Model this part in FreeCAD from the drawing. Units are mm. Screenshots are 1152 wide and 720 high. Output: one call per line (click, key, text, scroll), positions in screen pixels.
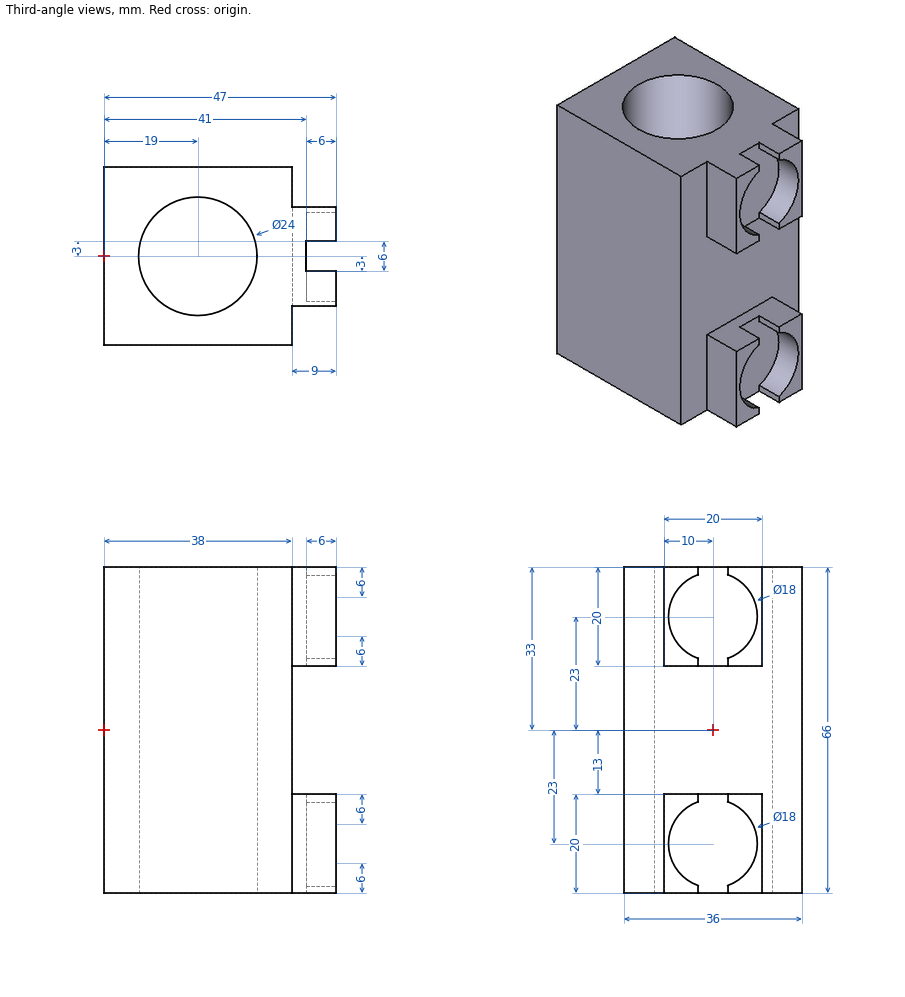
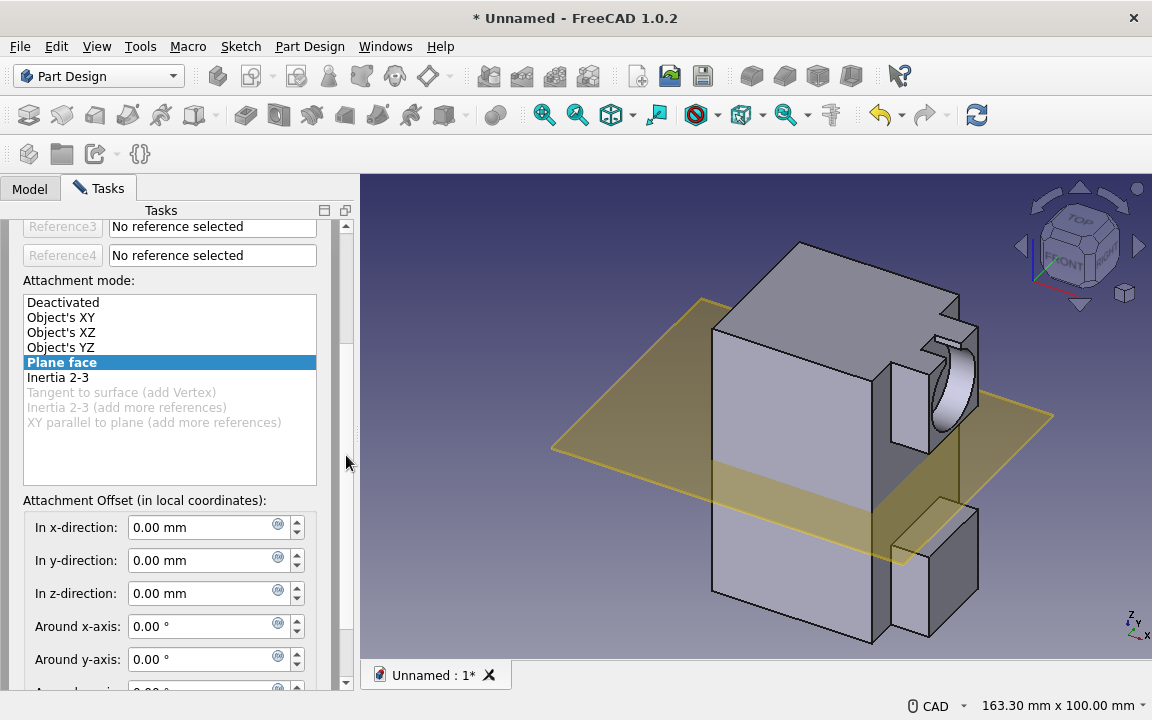
triple_click(210, 594)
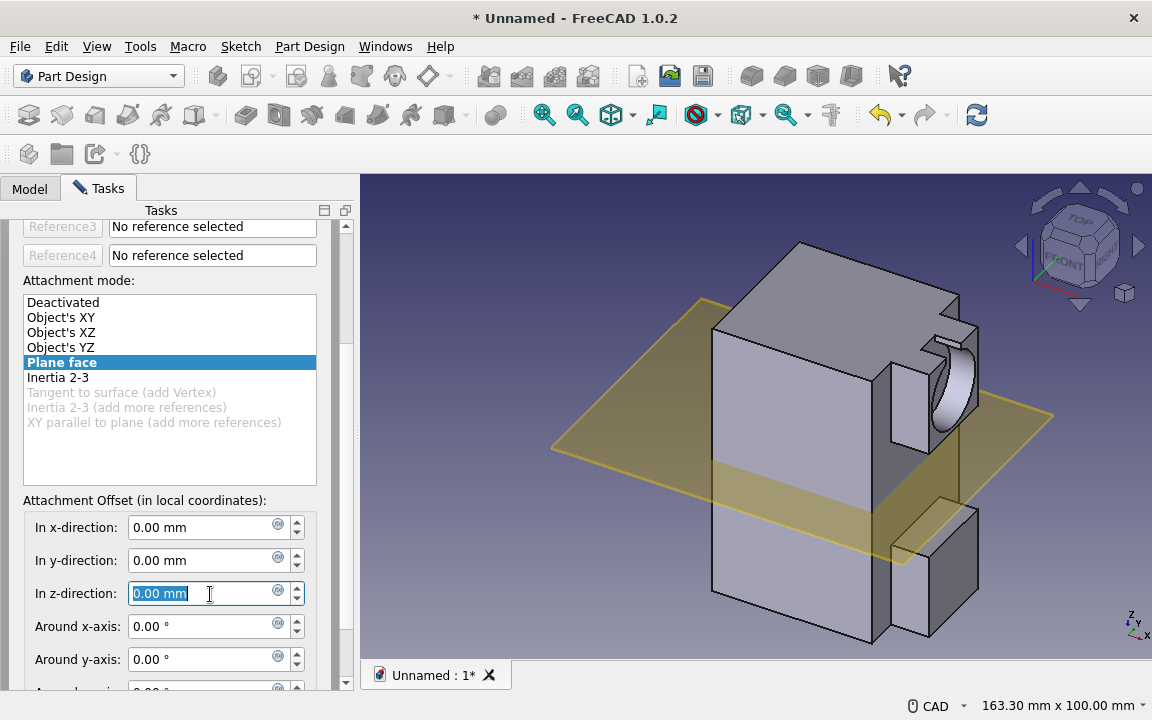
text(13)
key(Tab)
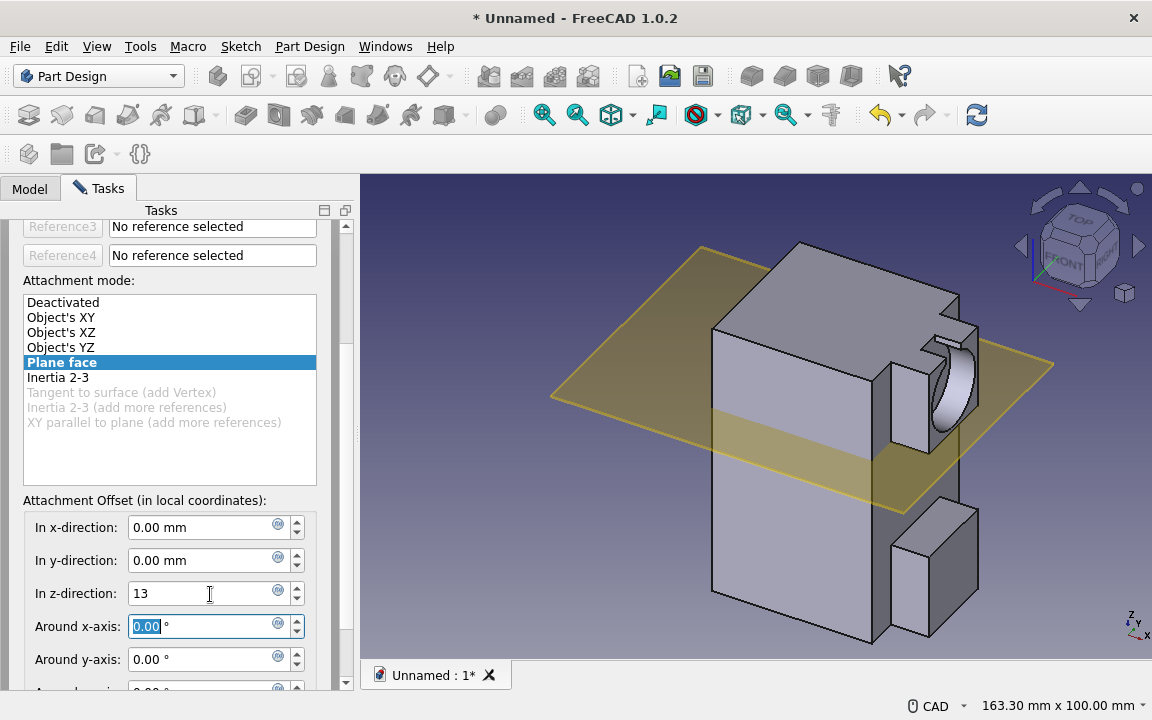
scroll(346, 455, up, 4)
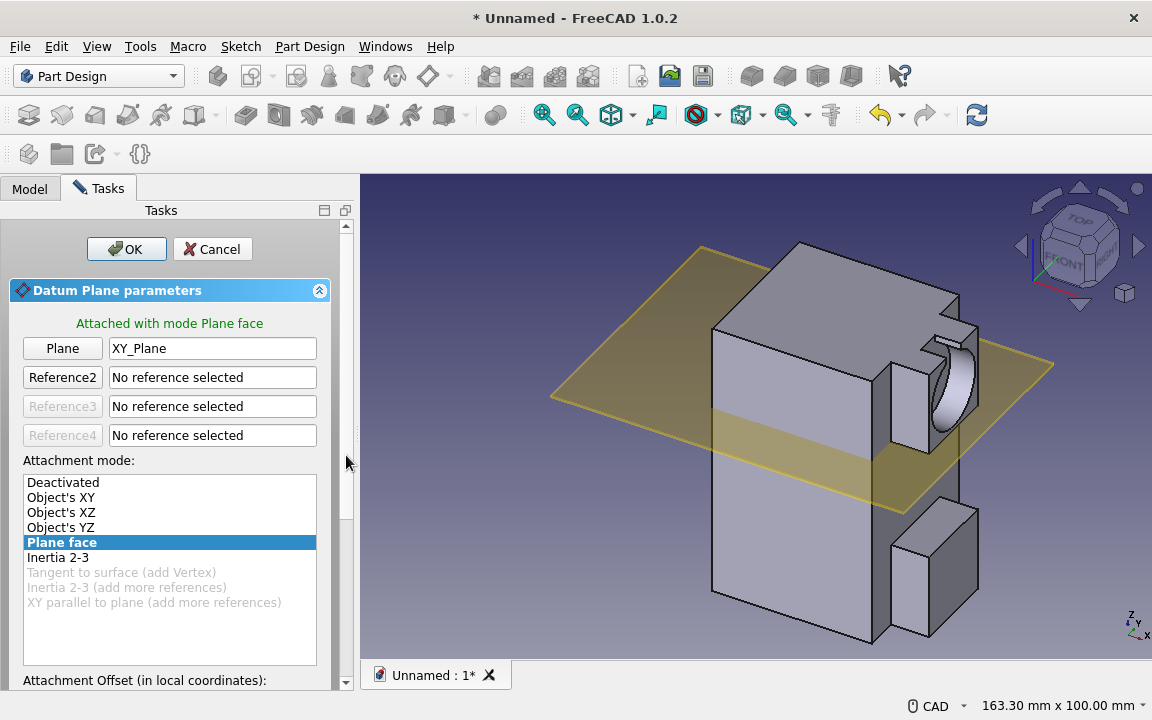
click(127, 249)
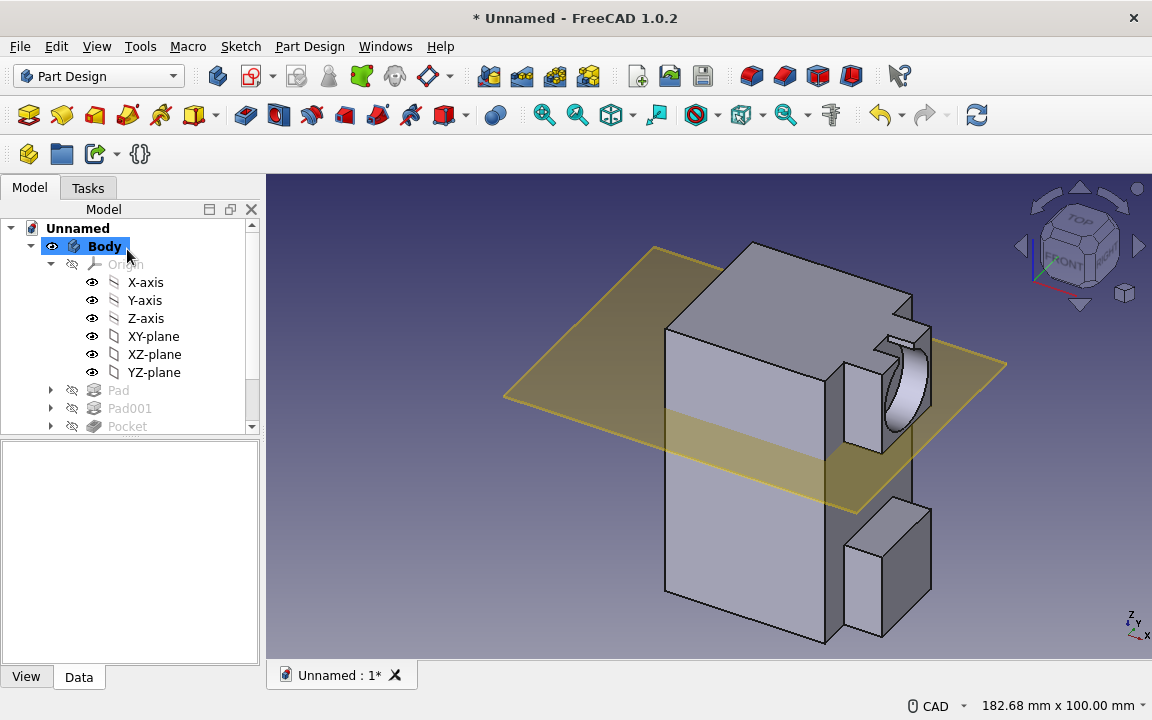
scroll(101, 332, down, 3)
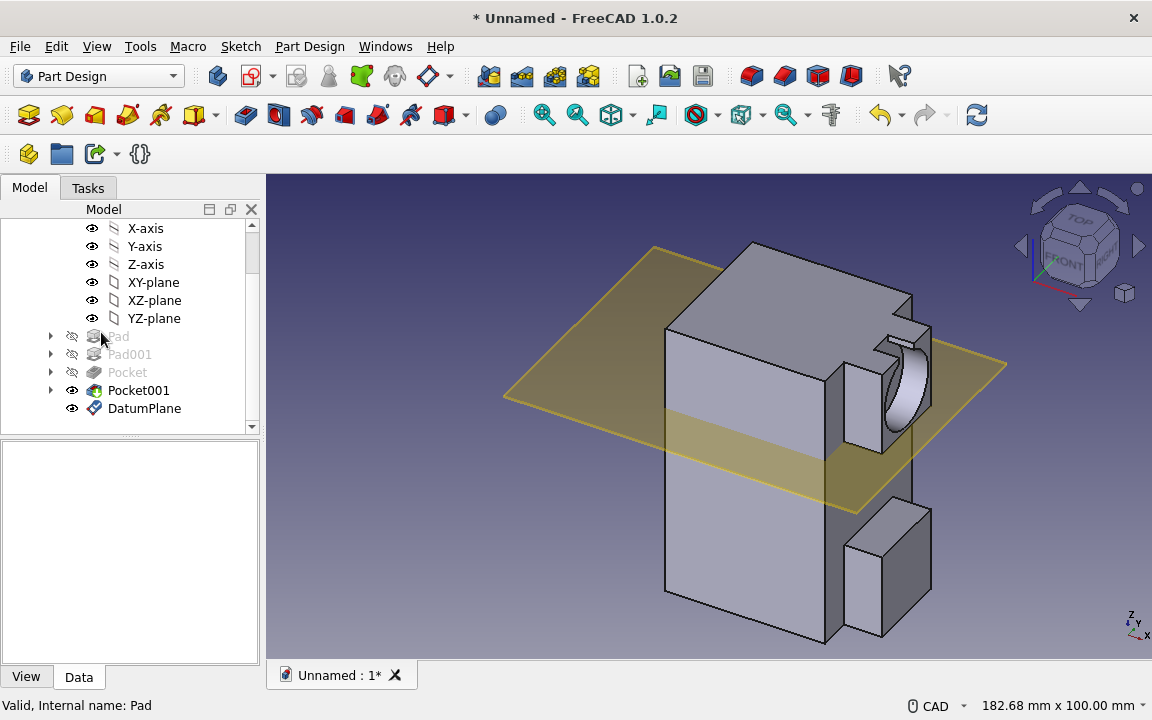
click(117, 408)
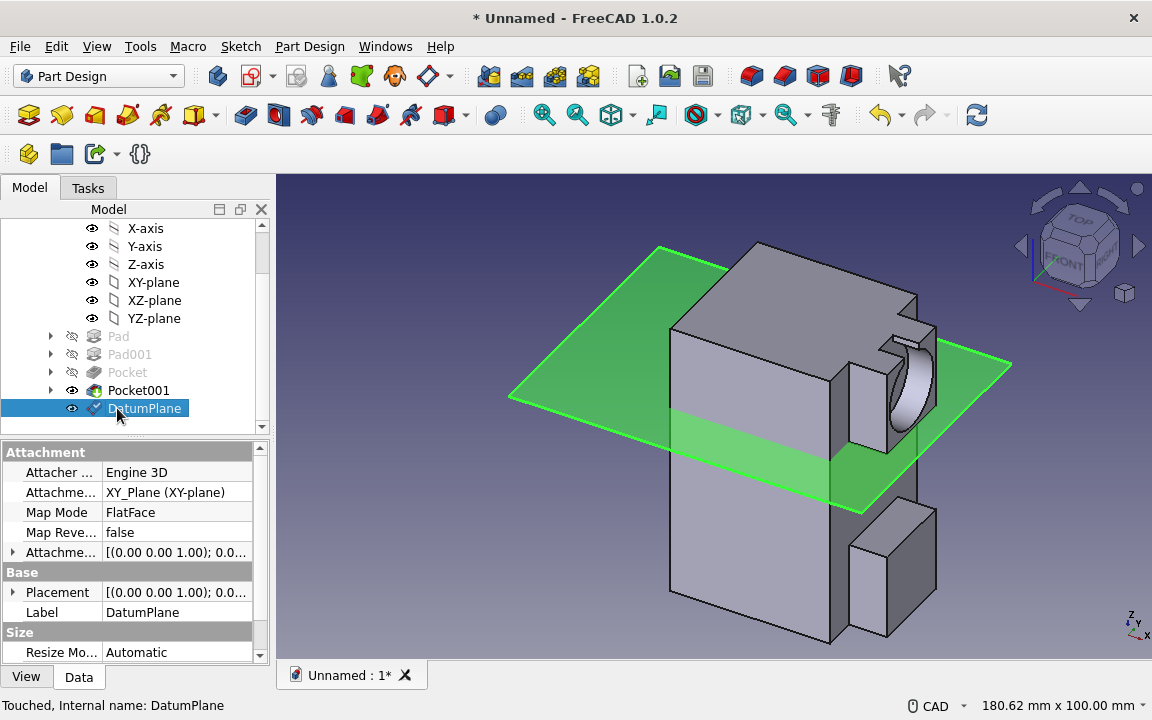
click(250, 76)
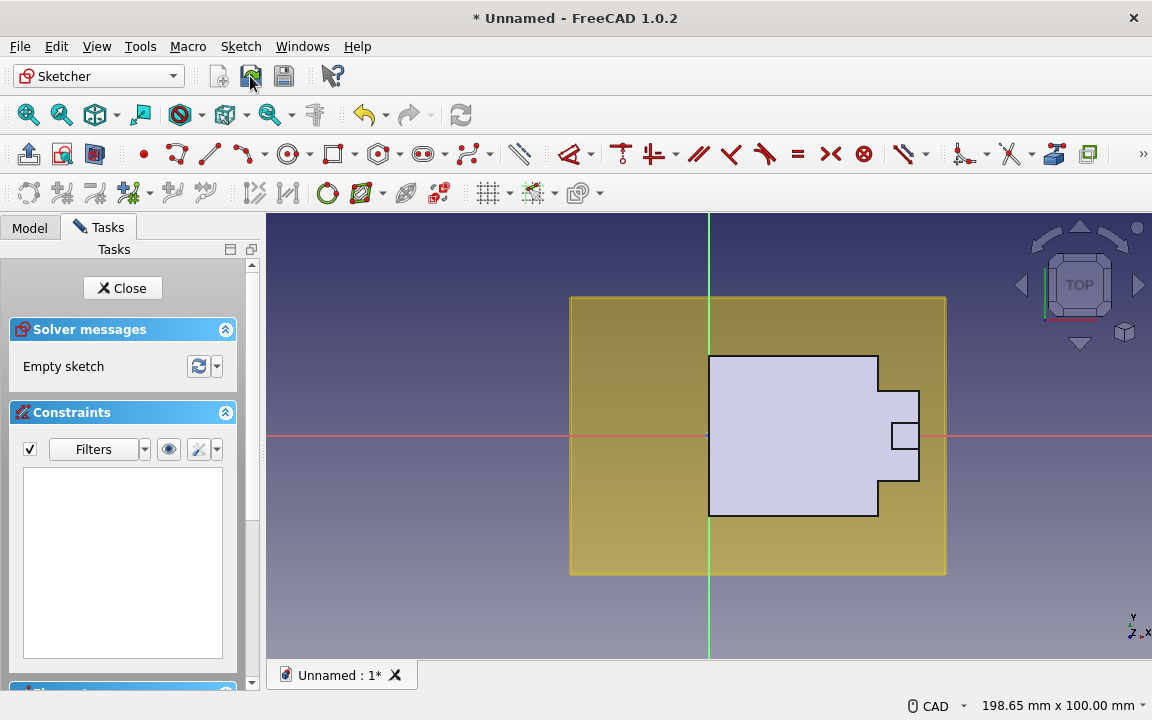
click(95, 154)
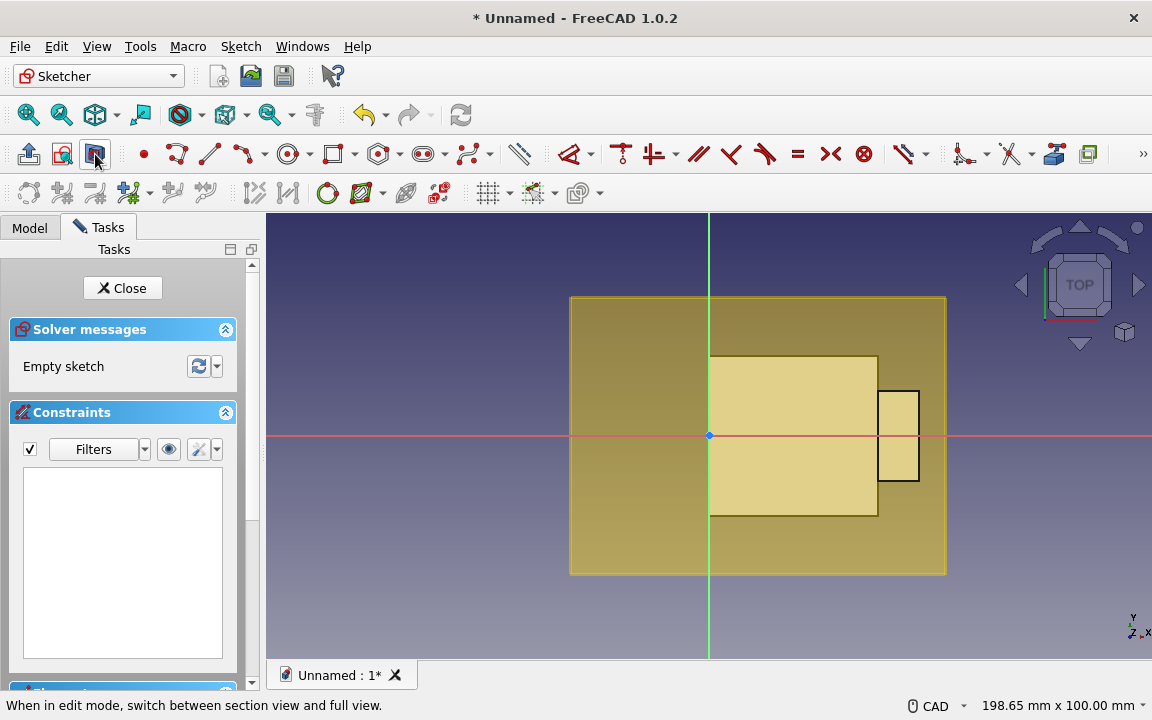
scroll(932, 436, up, 12)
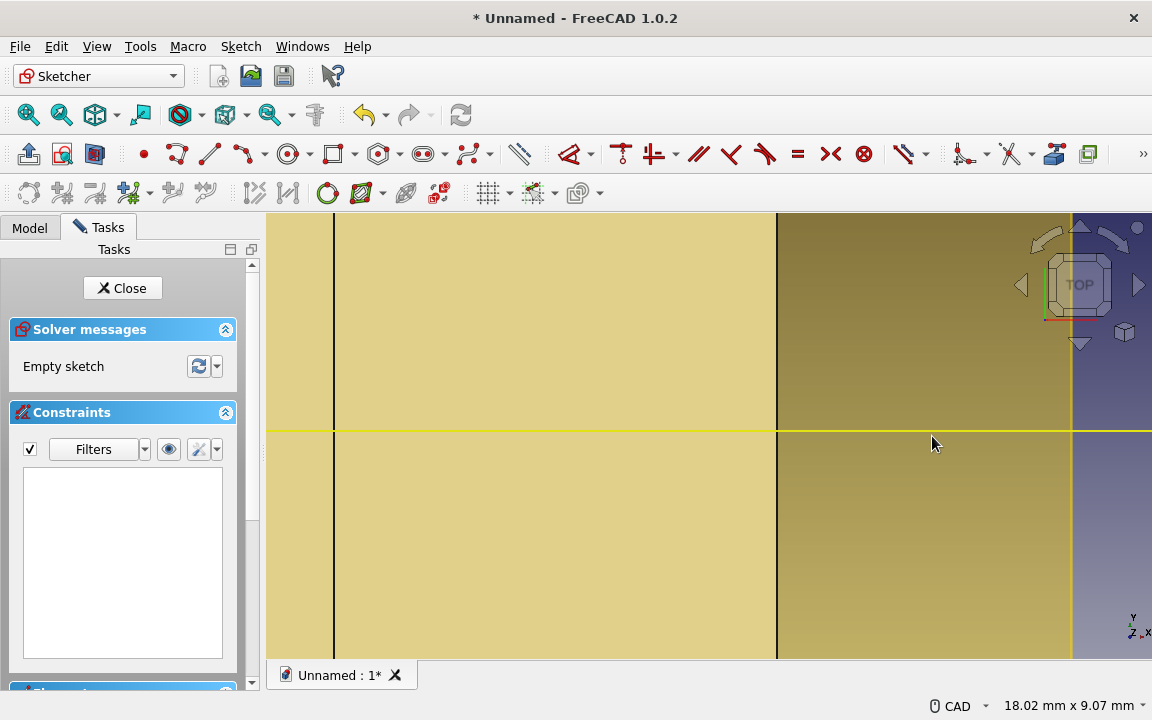
click(332, 154)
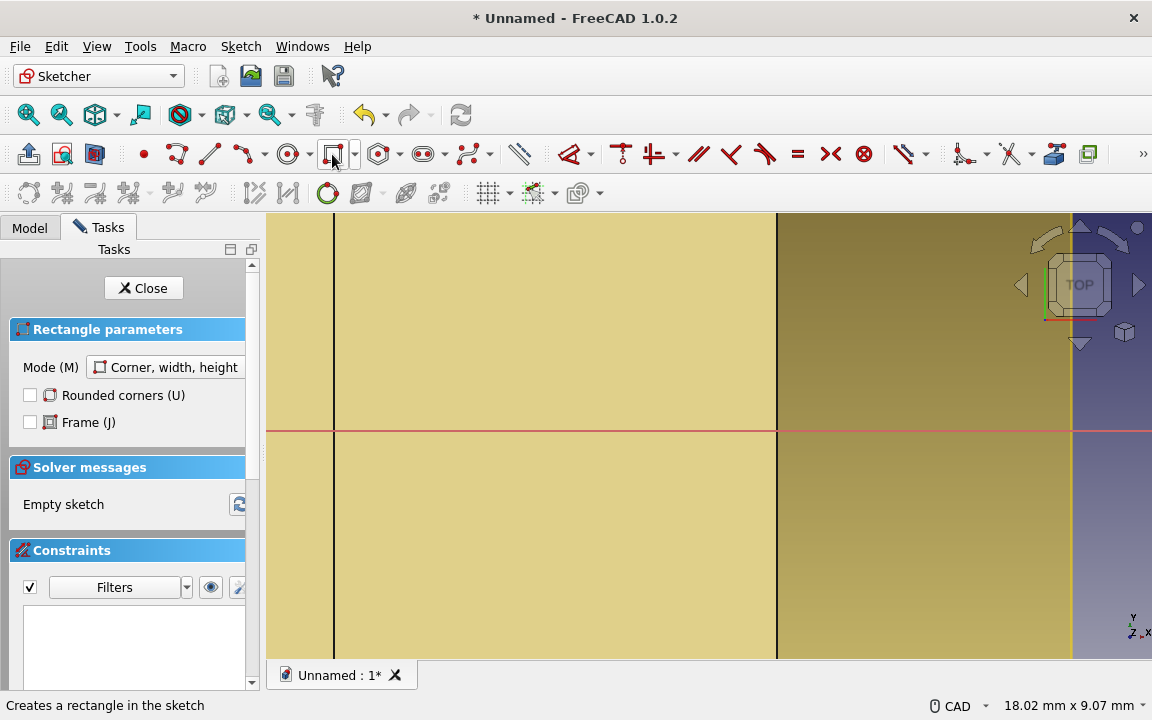
click(482, 283)
click(777, 578)
key(Escape)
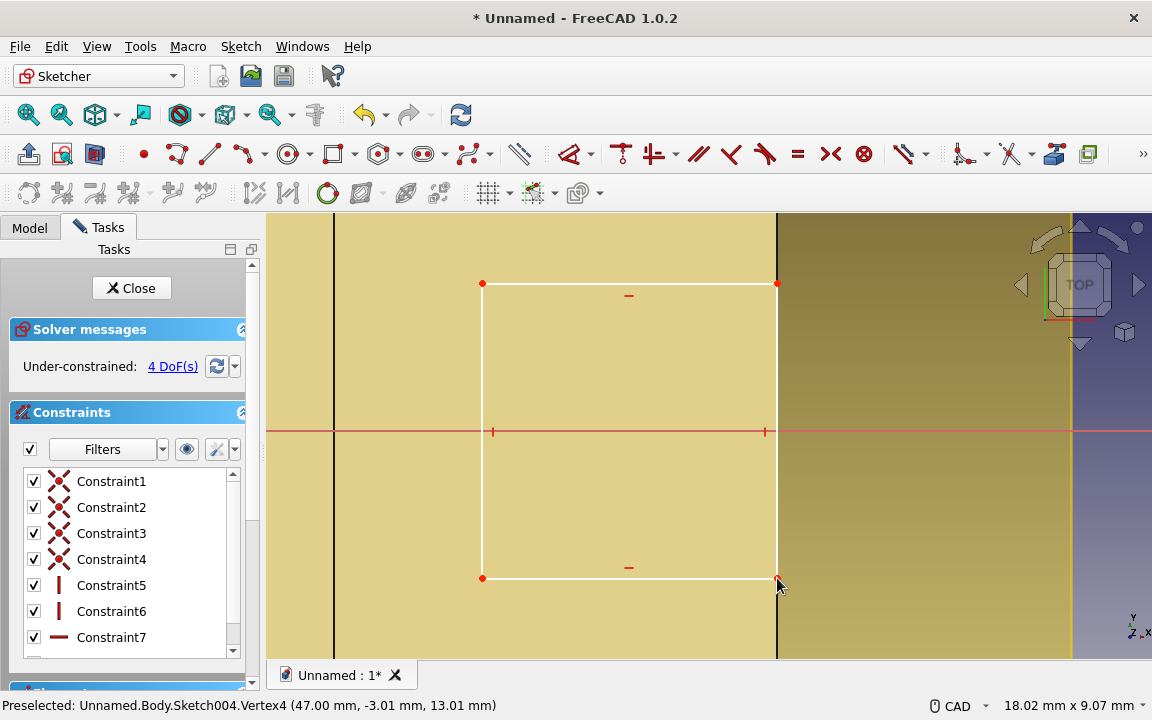
click(568, 154)